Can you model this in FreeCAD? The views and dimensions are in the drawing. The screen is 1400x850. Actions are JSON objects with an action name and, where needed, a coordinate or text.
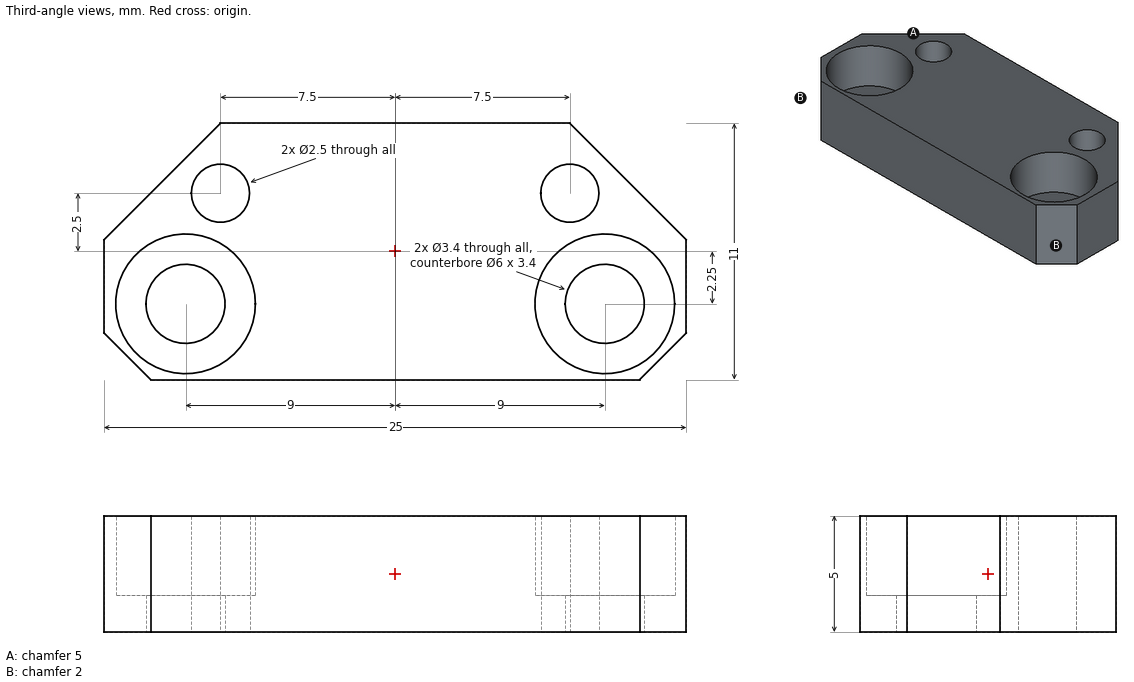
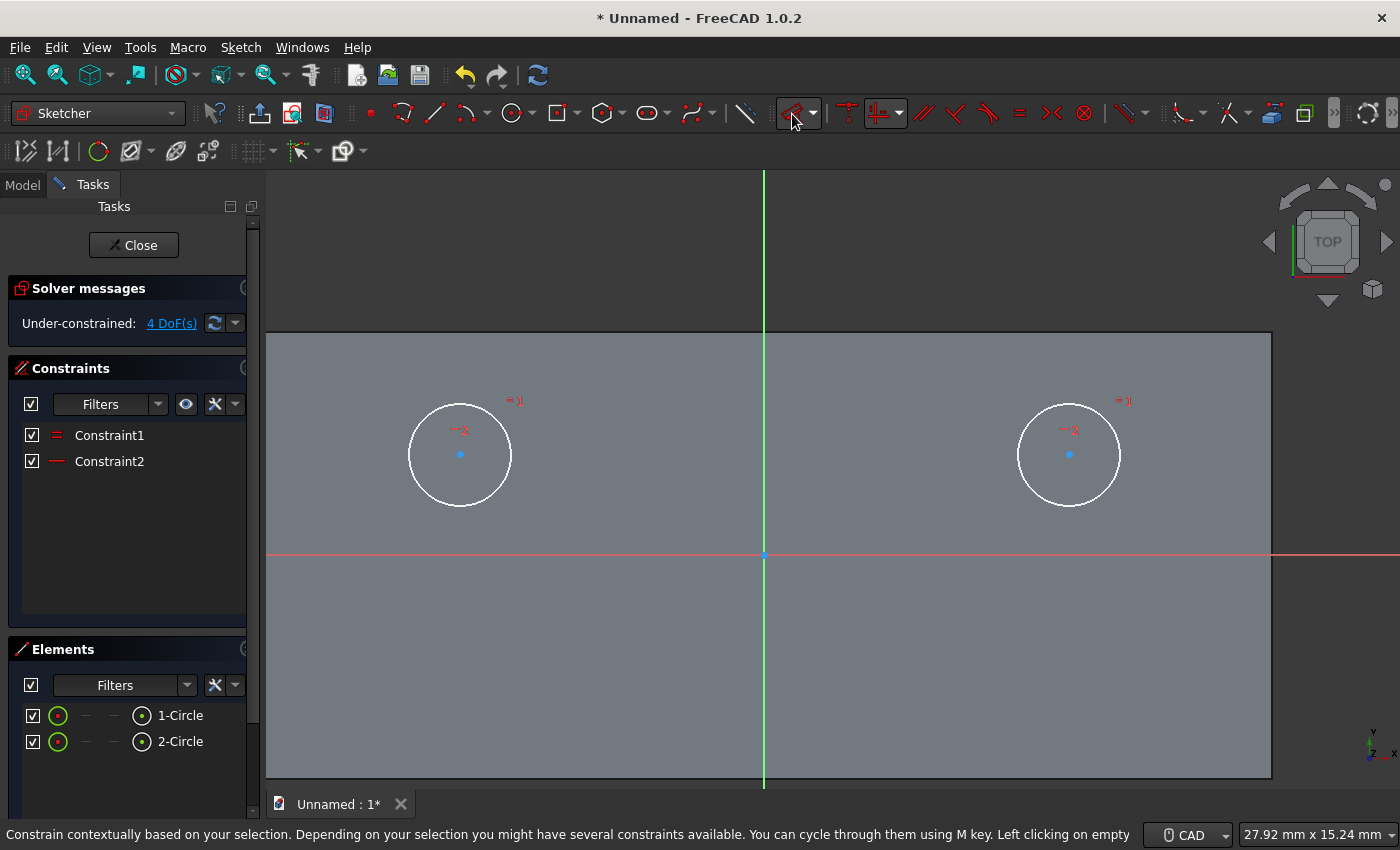
{"action": "left_click", "coordinate": [496, 419]}
{"action": "left_click", "coordinate": [519, 396]}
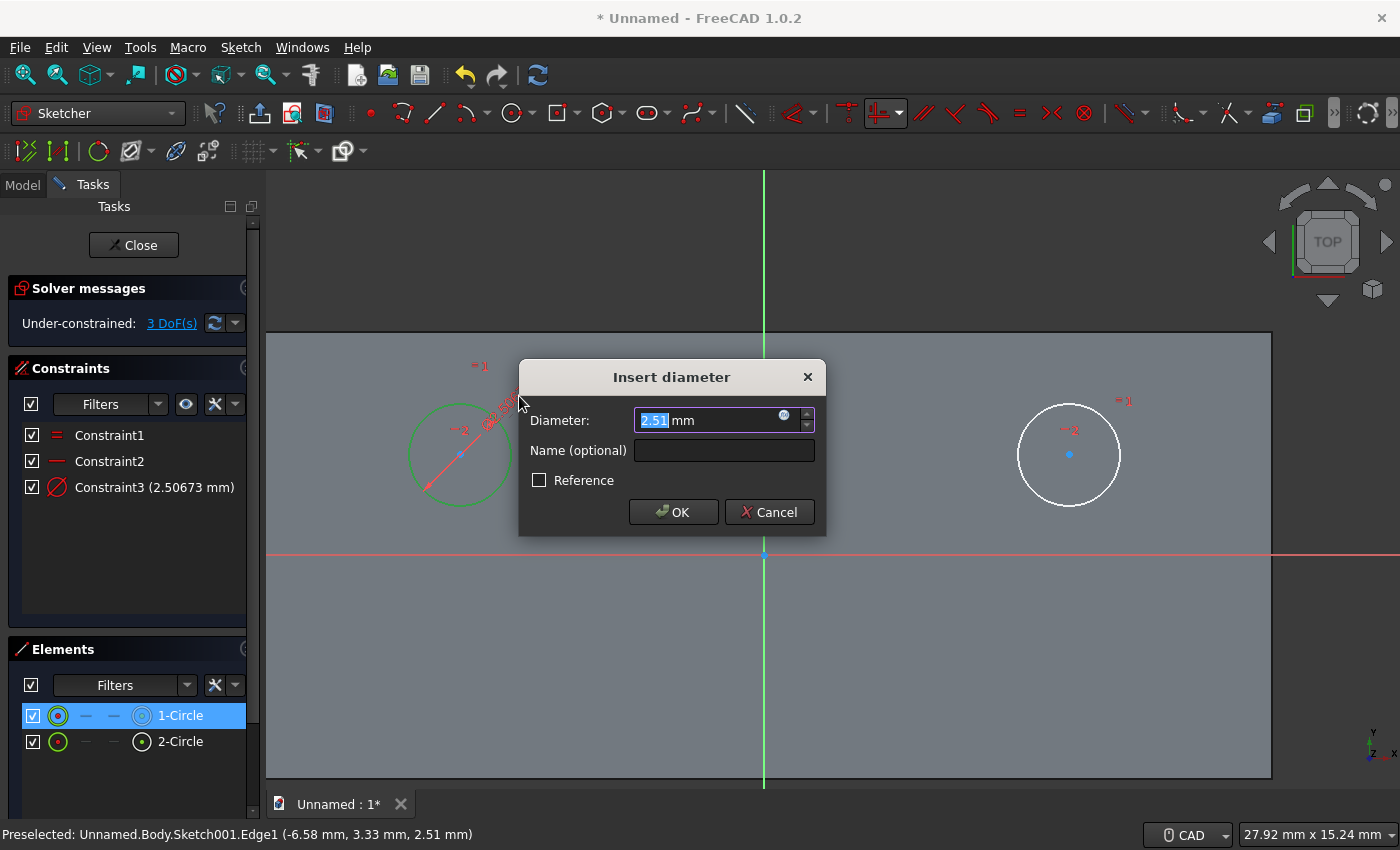
{"action": "type", "text": "2.5"}
{"action": "key", "text": "Return"}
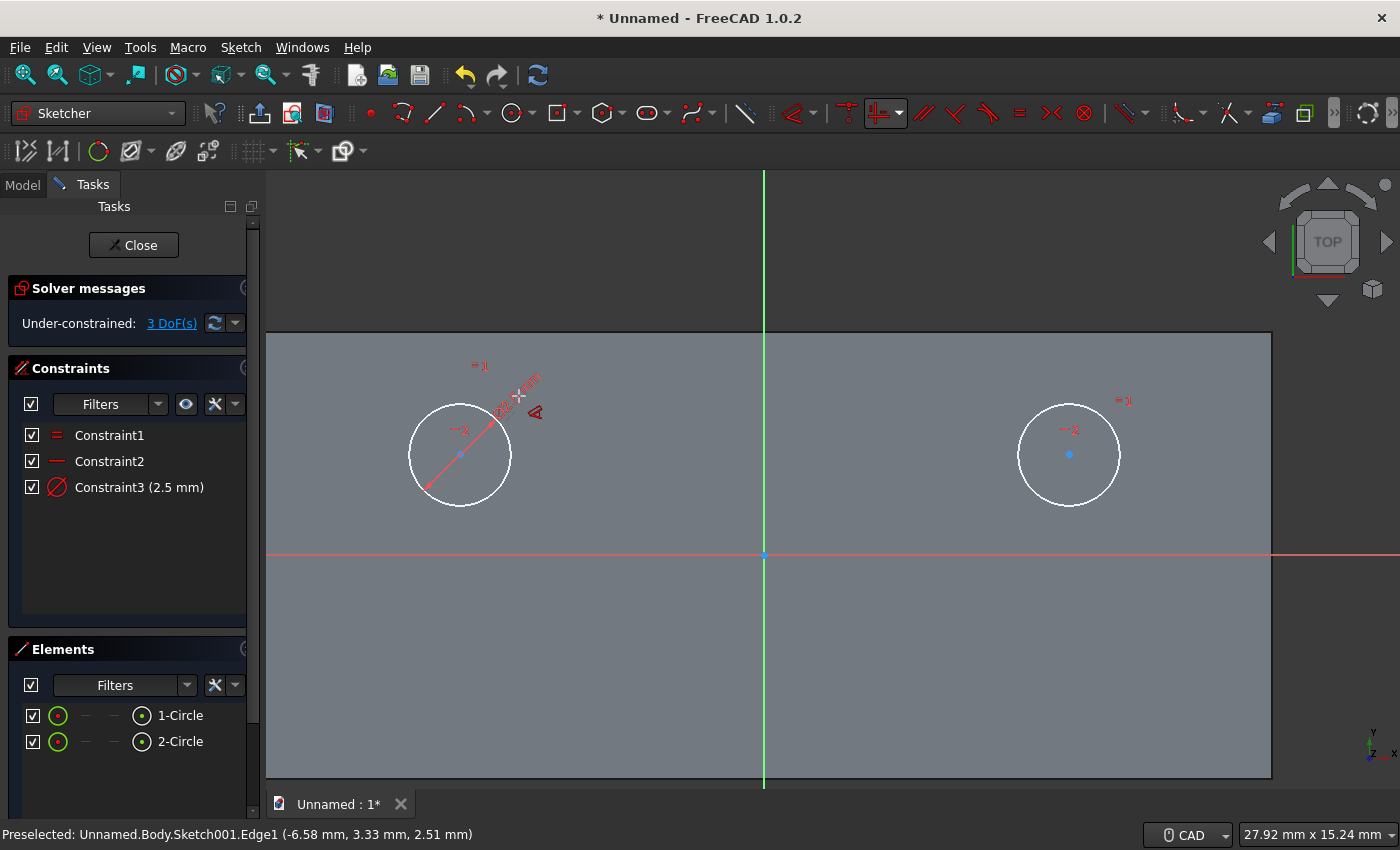
{"action": "left_click", "coordinate": [460, 455]}
{"action": "left_click", "coordinate": [612, 589]}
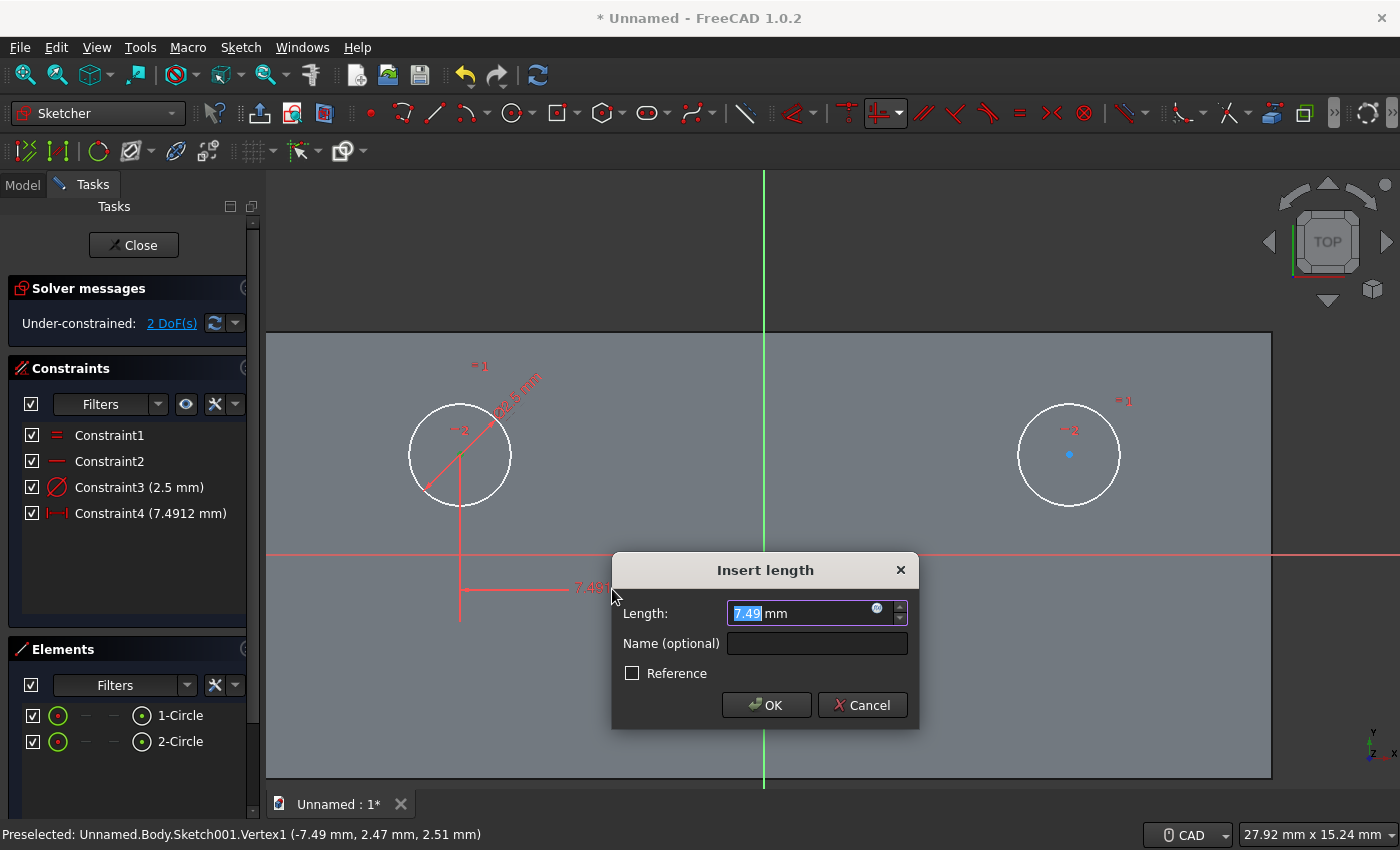
{"action": "type", "text": "7.5"}
{"action": "key", "text": "Return"}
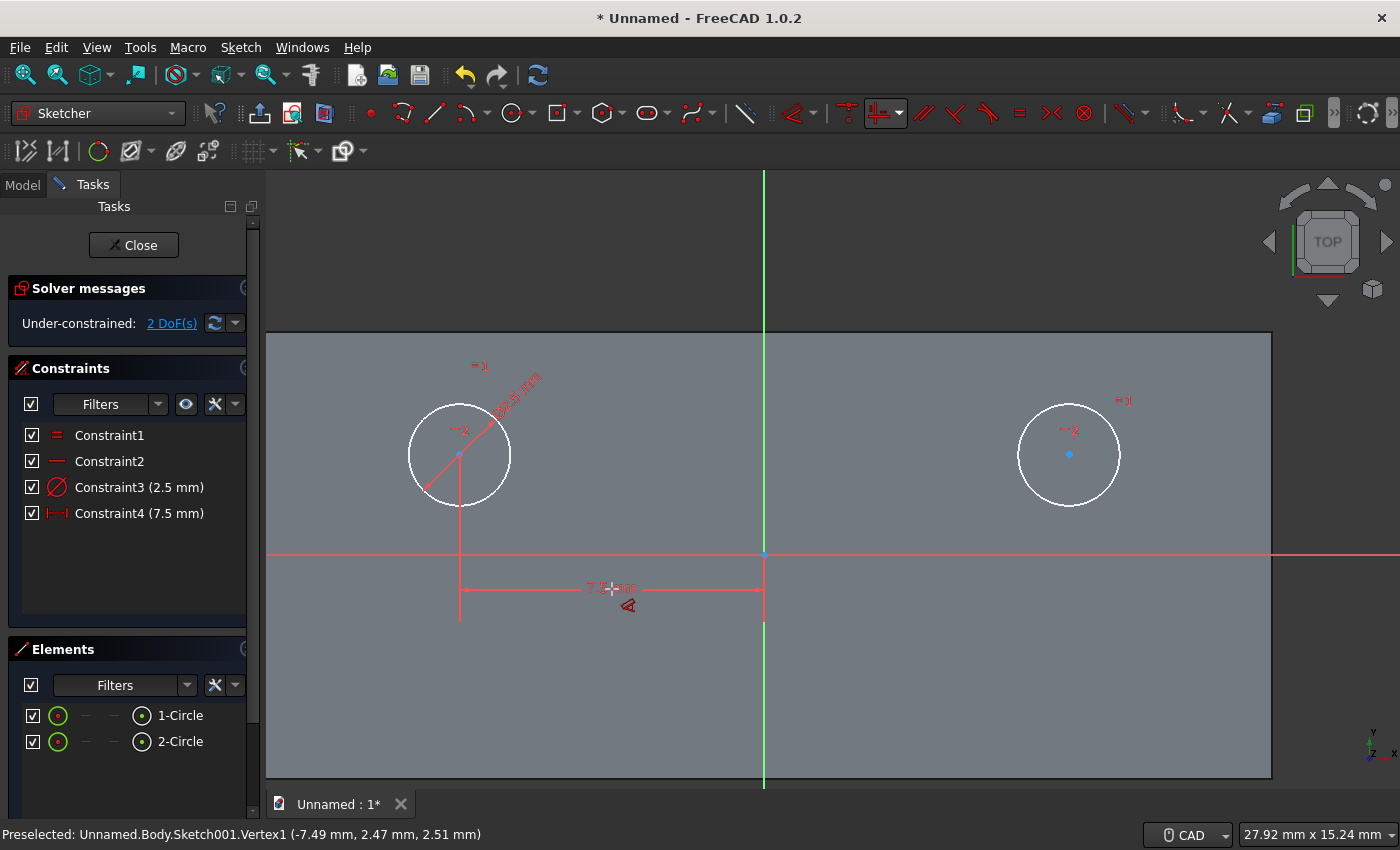
{"action": "left_click", "coordinate": [460, 455]}
{"action": "left_click", "coordinate": [426, 528]}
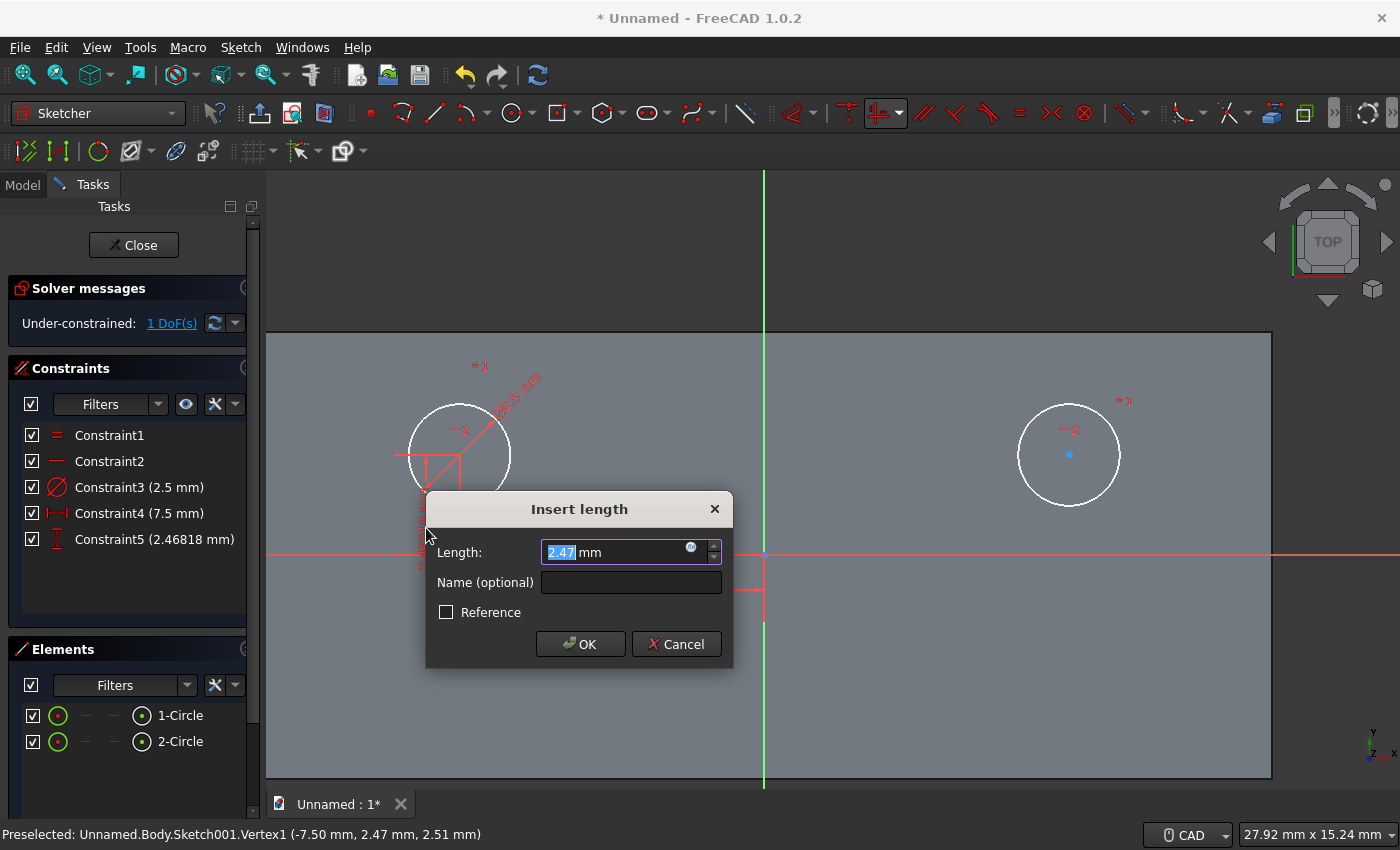
{"action": "type", "text": "2.5"}
{"action": "key", "text": "Return"}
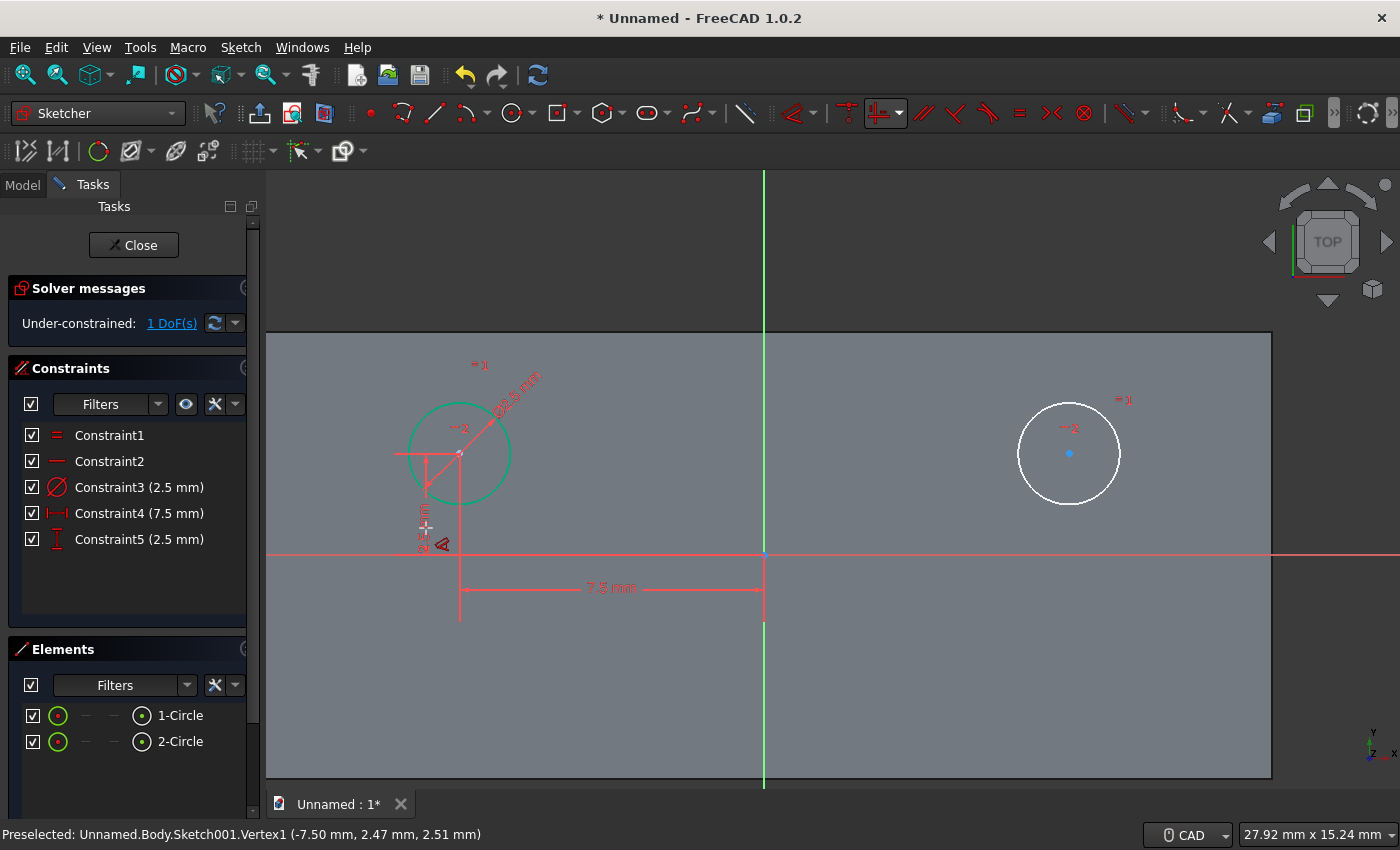
{"action": "left_click", "coordinate": [1069, 454]}
{"action": "left_click", "coordinate": [917, 589]}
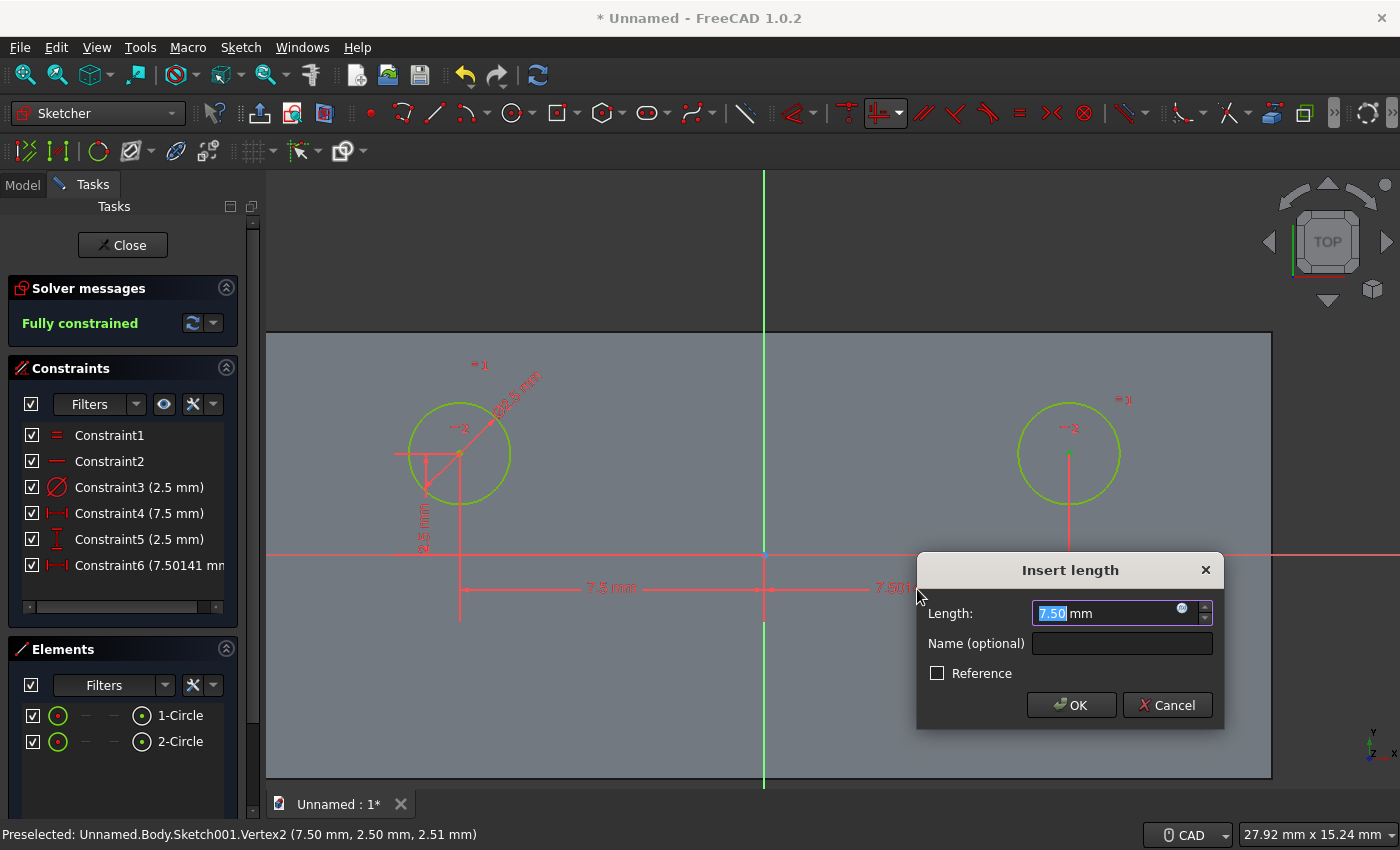
{"action": "type", "text": "7.5"}
{"action": "key", "text": "Return"}
{"action": "key", "text": "Escape"}